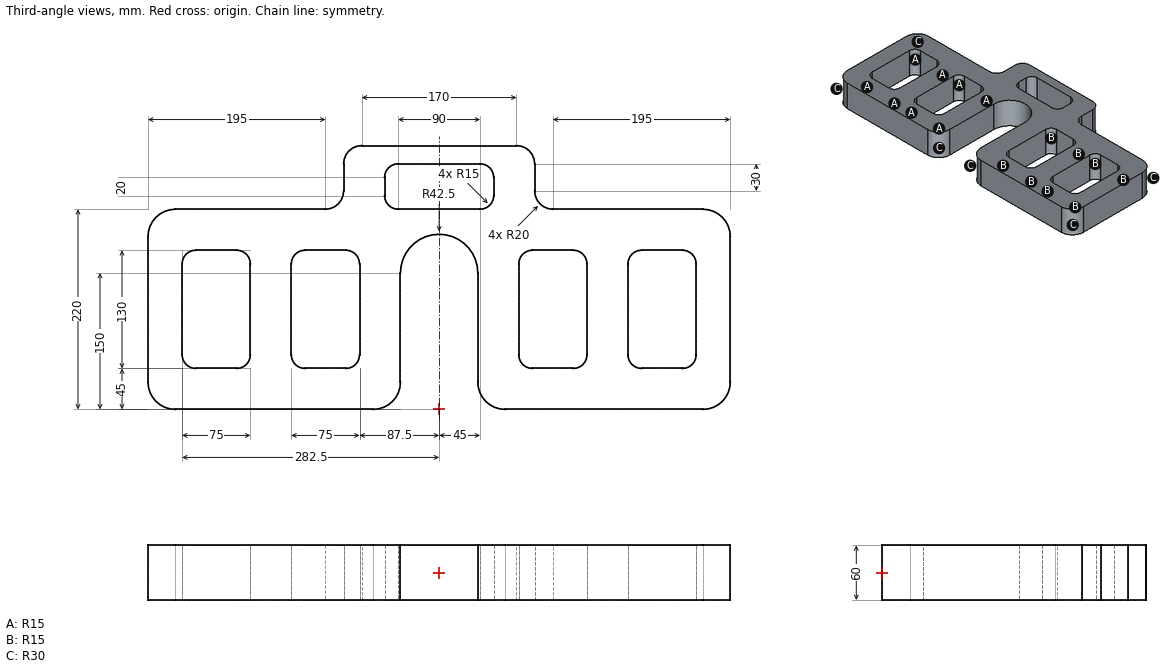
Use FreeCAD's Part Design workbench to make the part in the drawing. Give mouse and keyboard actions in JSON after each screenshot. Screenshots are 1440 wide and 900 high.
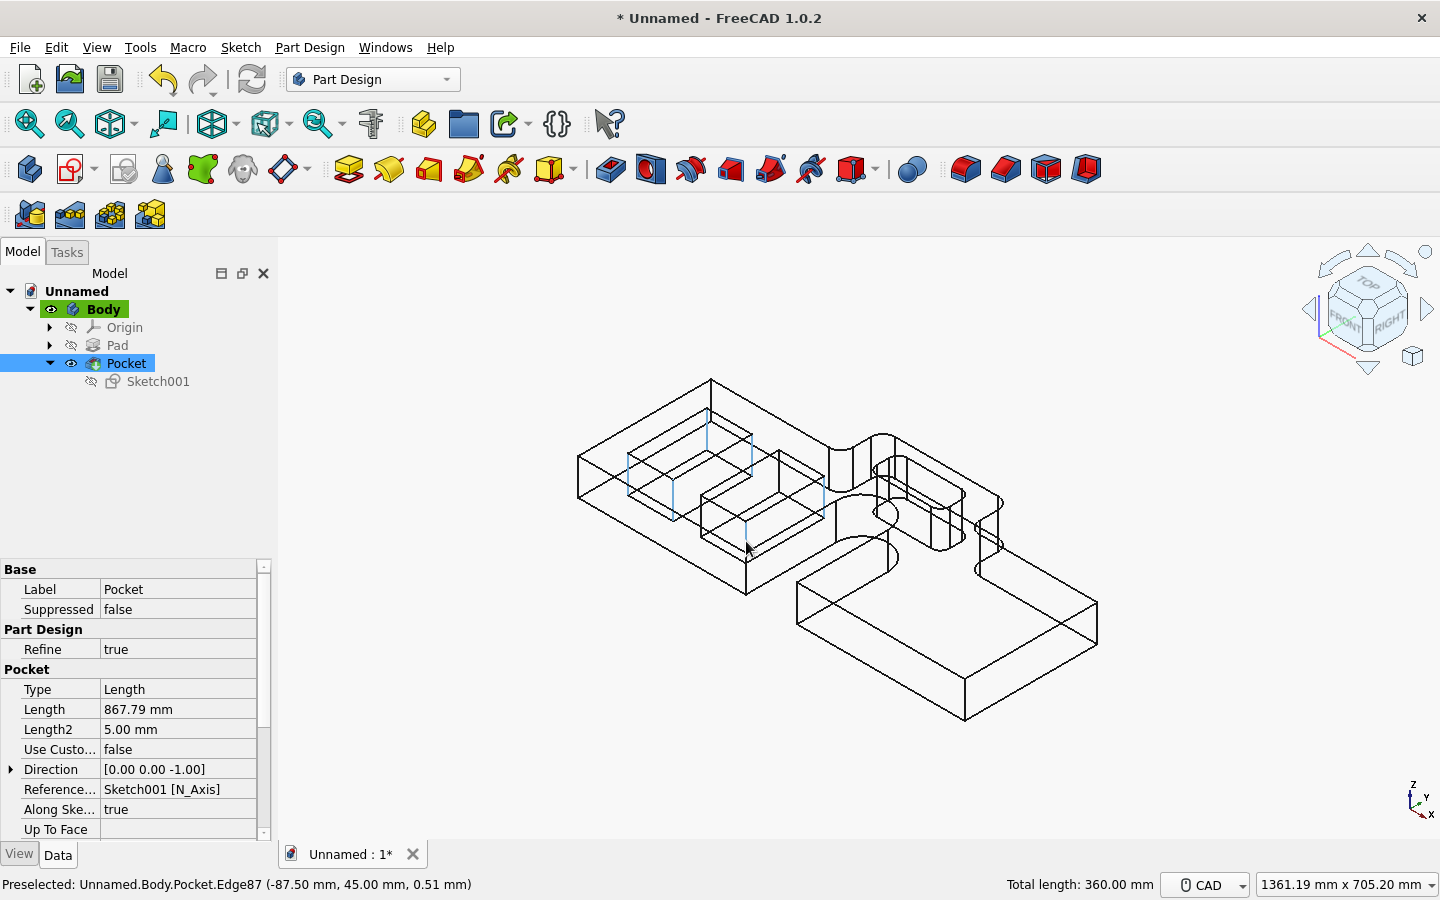
{"action": "left_click", "coordinate": [701, 515], "text": "ctrl"}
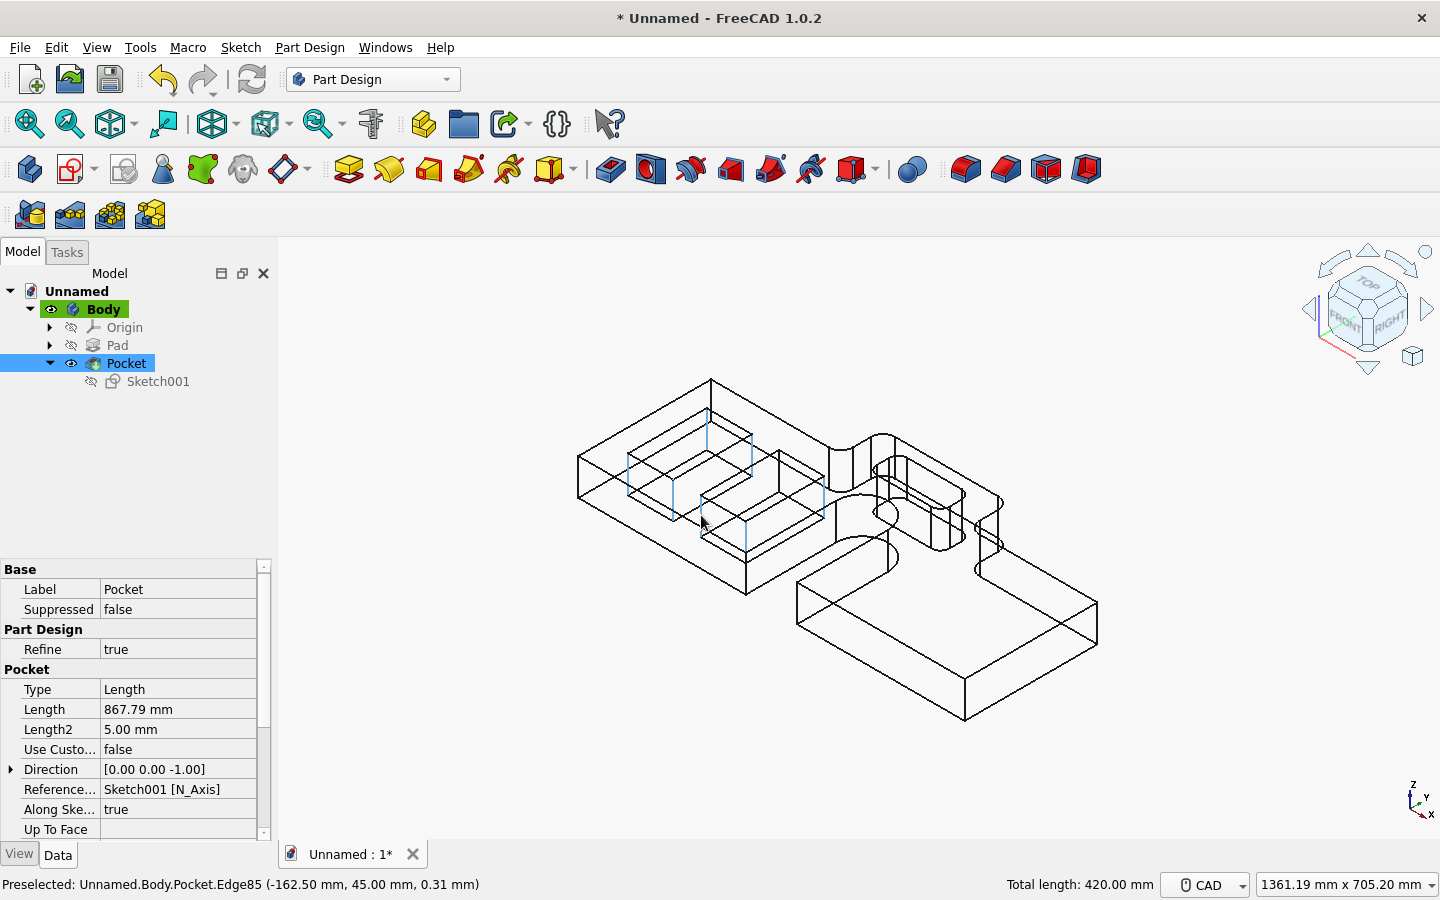
{"action": "left_click", "coordinate": [779, 470], "text": "ctrl"}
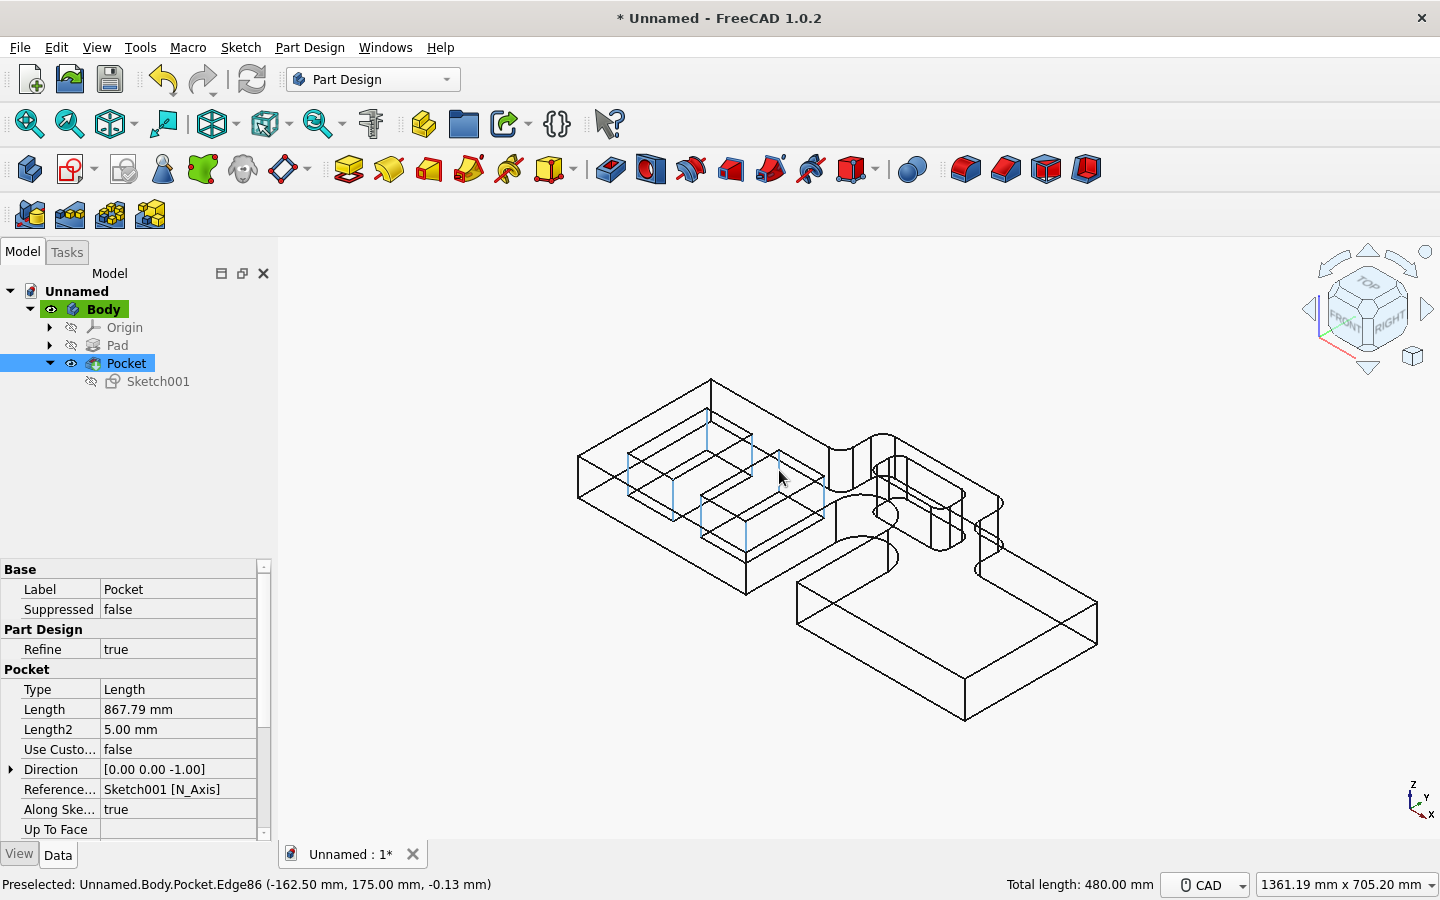
{"action": "key", "text": "v 1"}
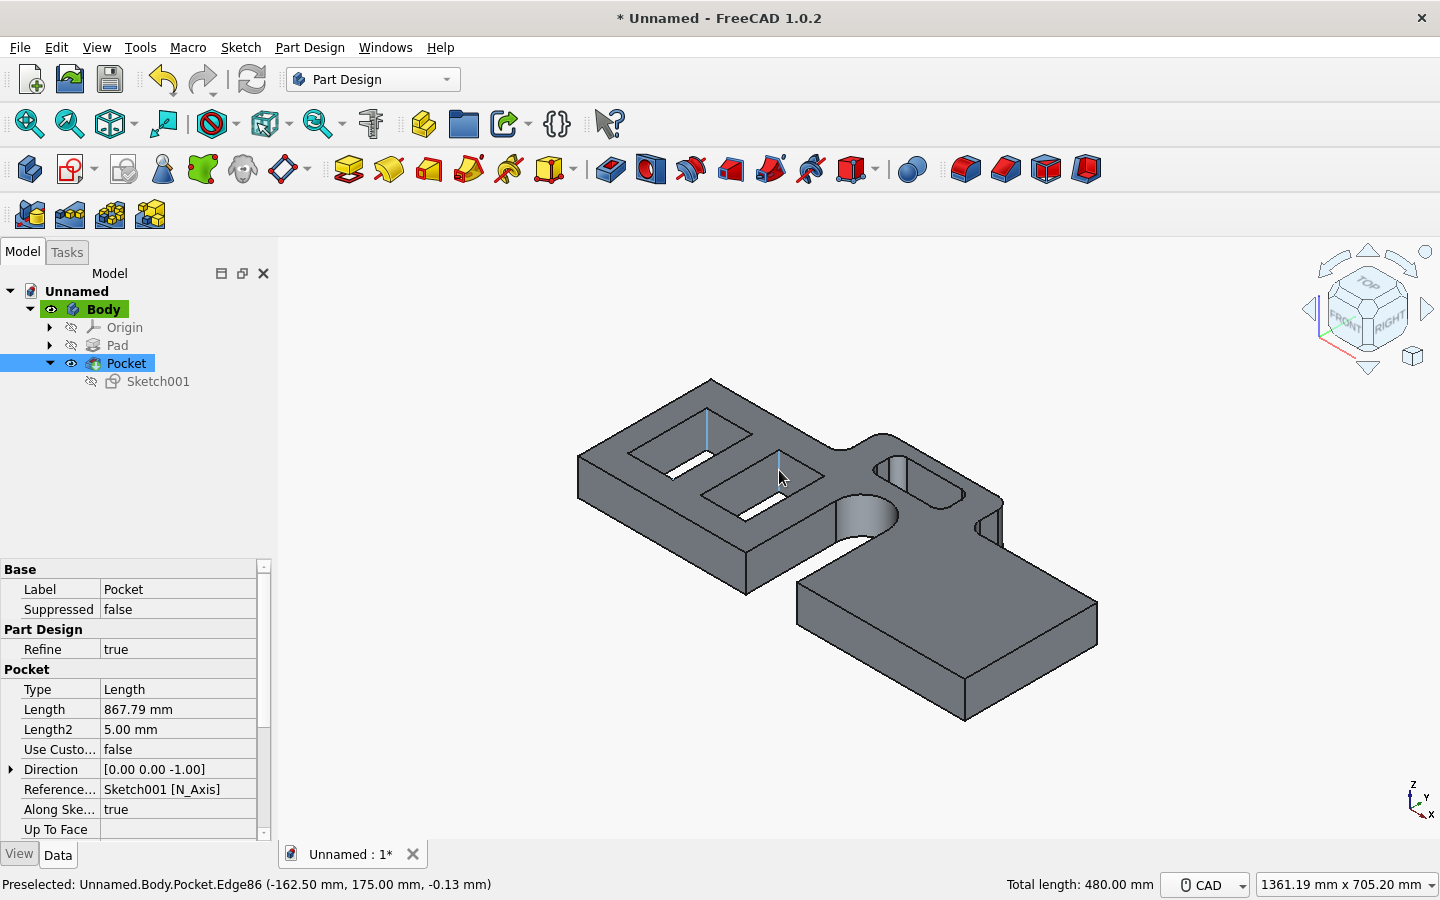
{"action": "left_click", "coordinate": [966, 170]}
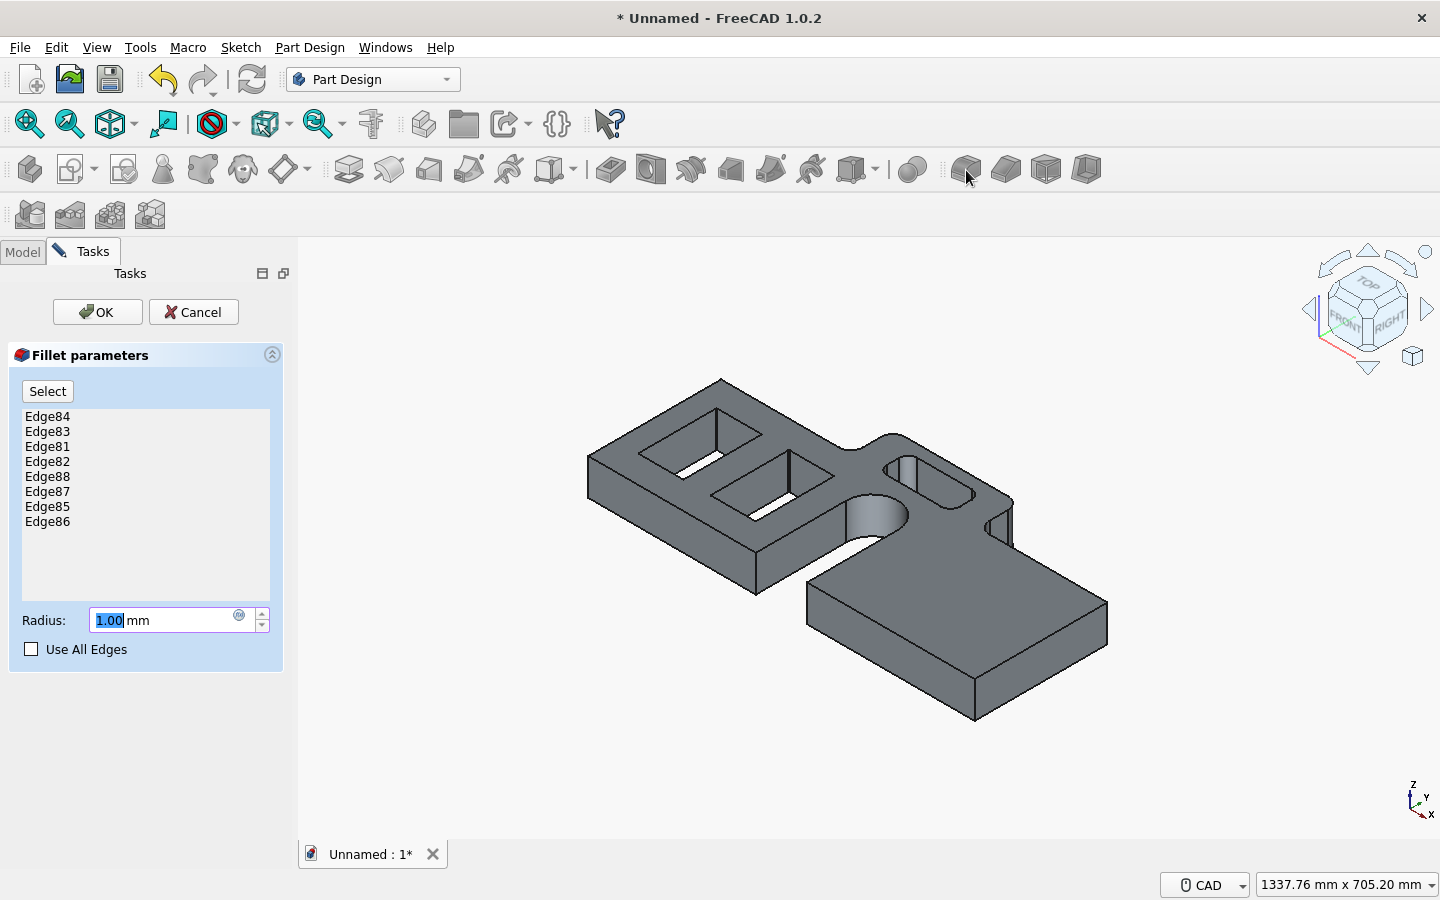
{"action": "type", "text": "15"}
{"action": "key", "text": "Tab"}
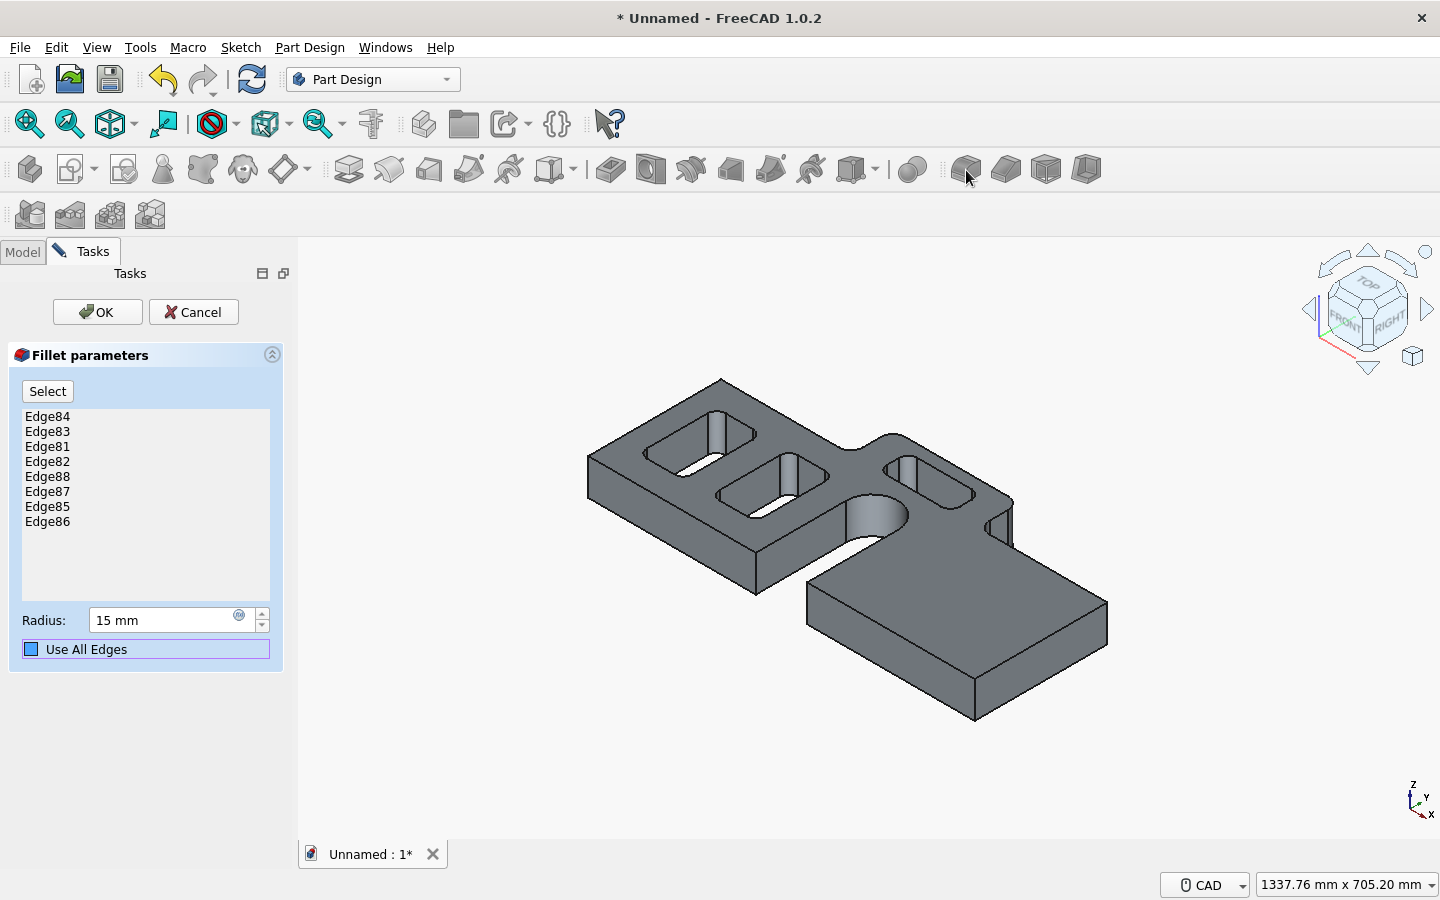
{"action": "left_click", "coordinate": [98, 312]}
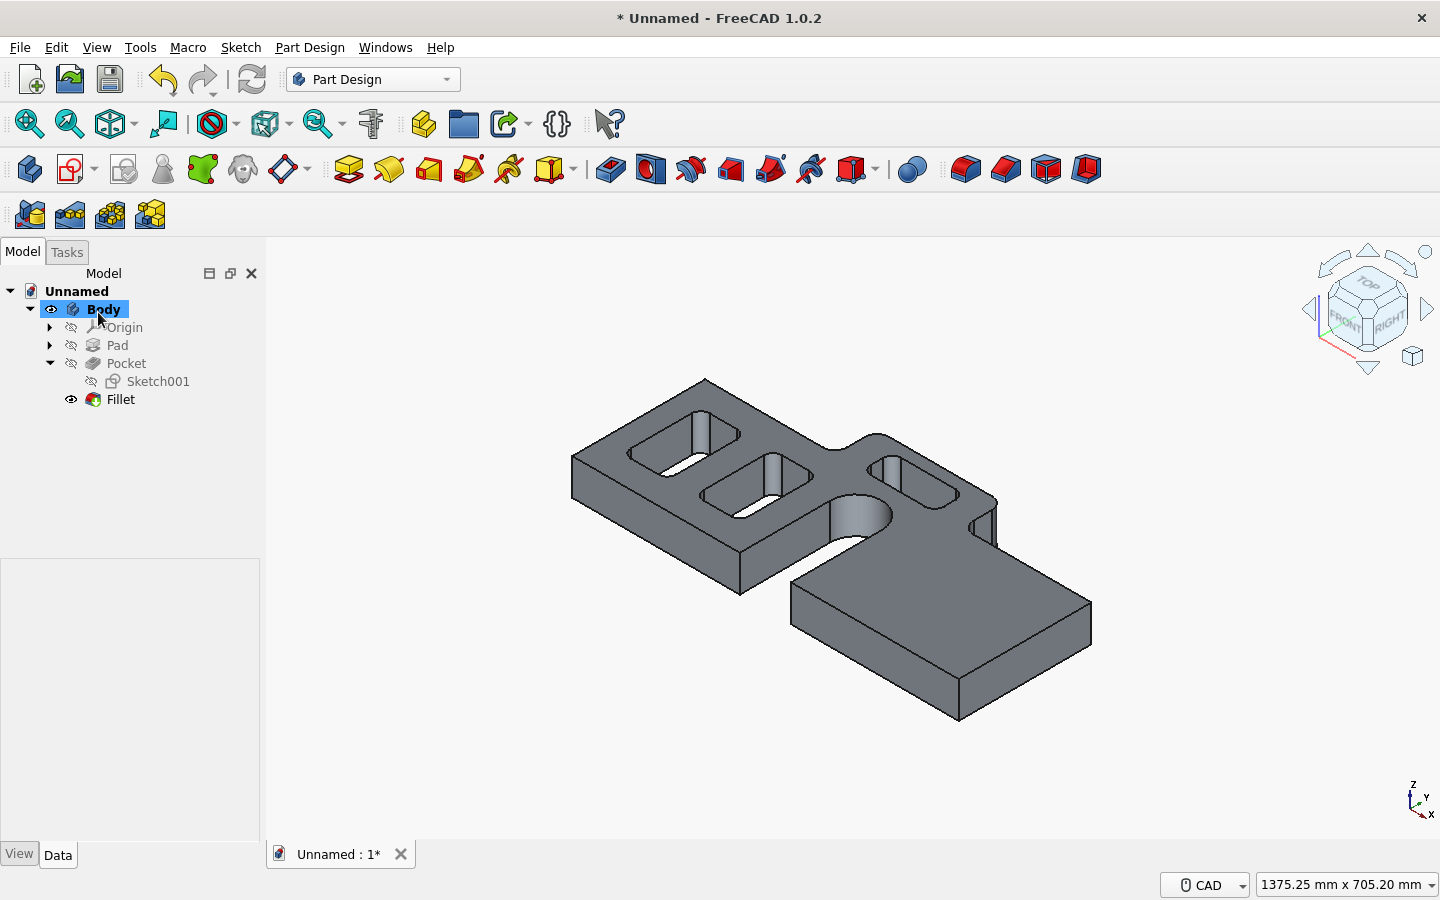
{"action": "left_click", "coordinate": [116, 363]}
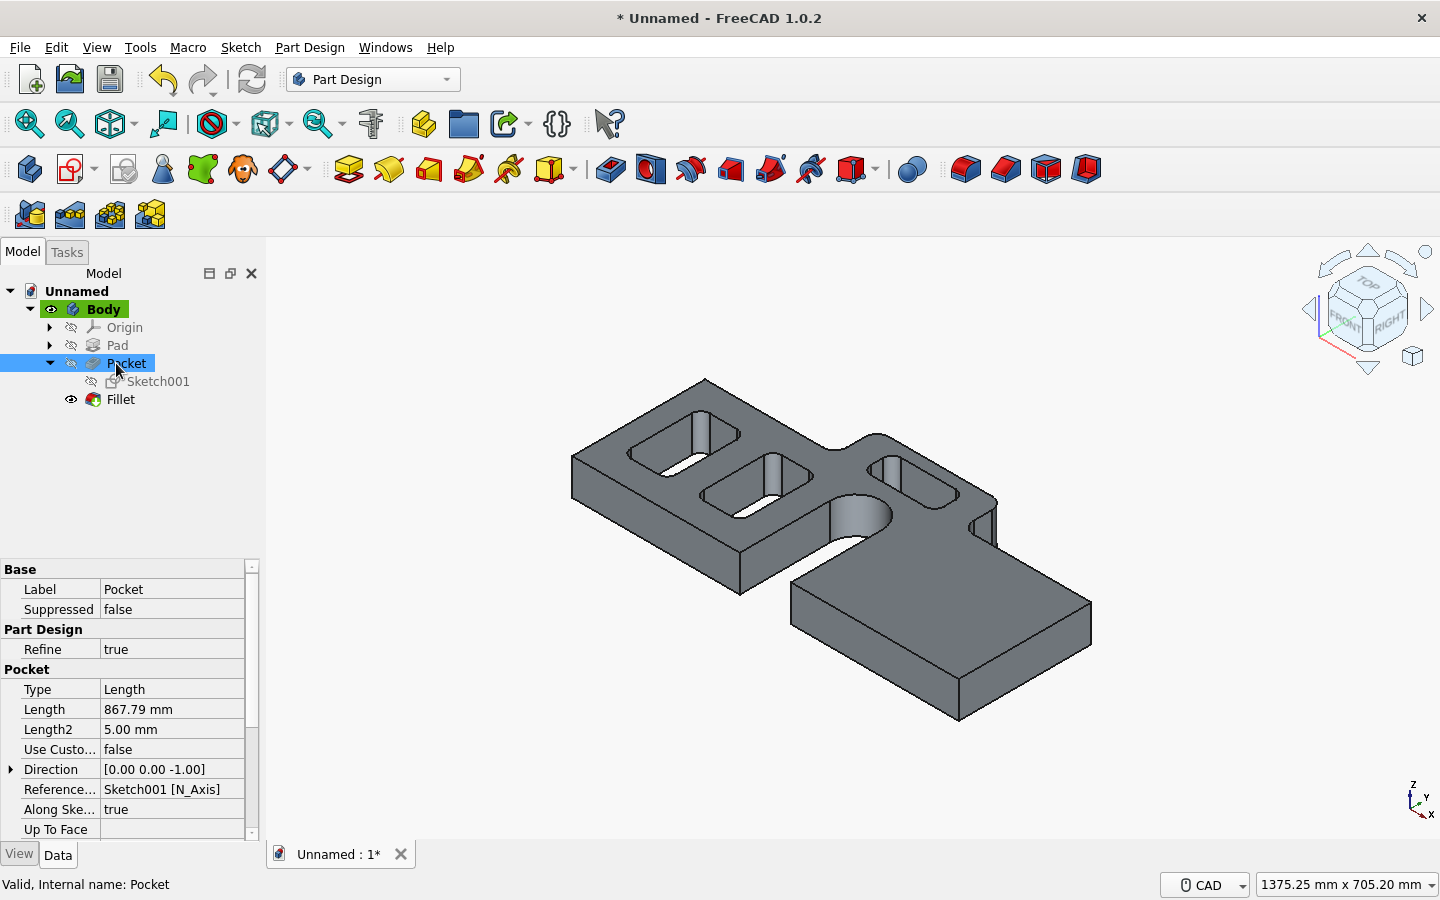
{"action": "left_click", "coordinate": [30, 214]}